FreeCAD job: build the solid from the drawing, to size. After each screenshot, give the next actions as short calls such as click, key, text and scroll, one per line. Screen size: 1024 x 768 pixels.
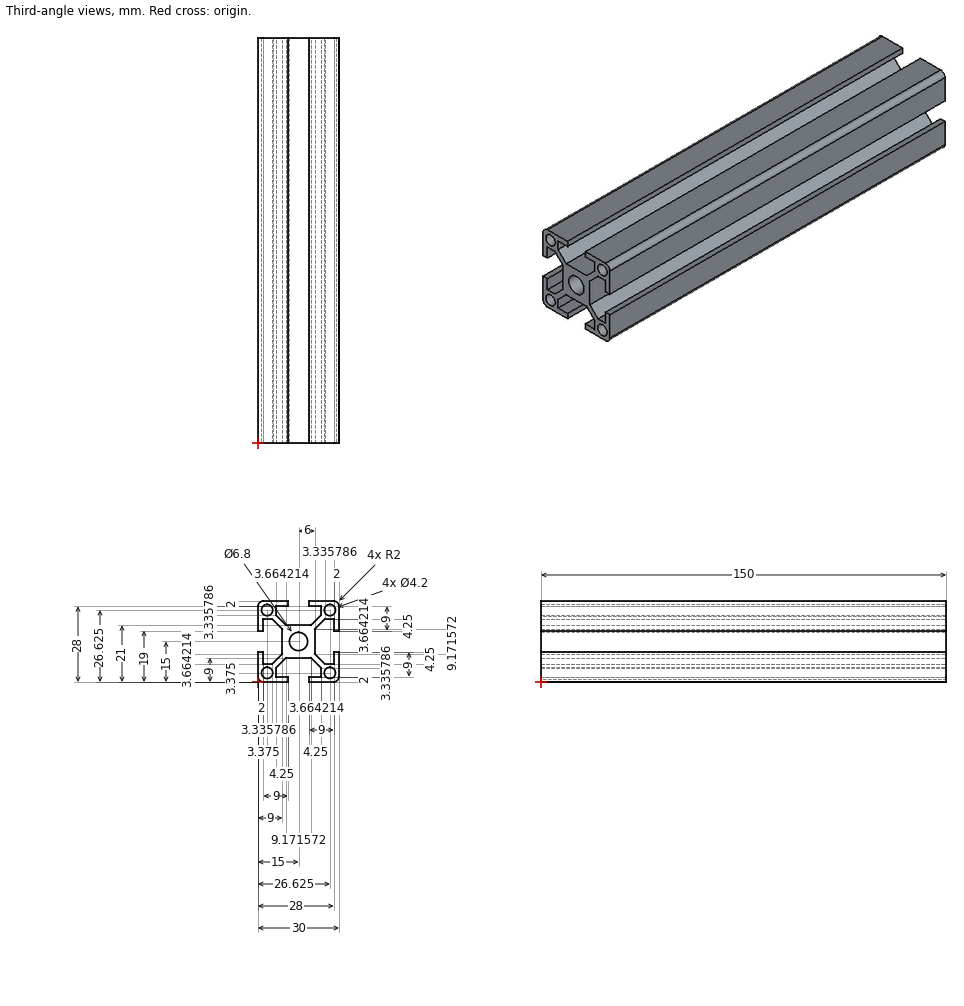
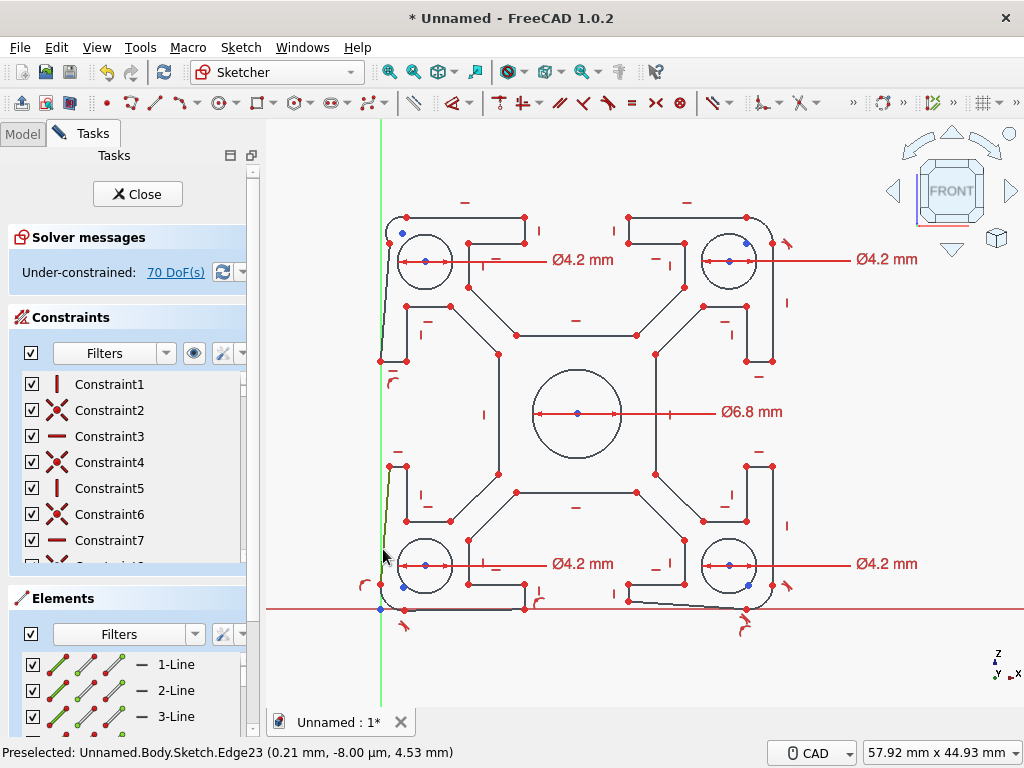
click(382, 596)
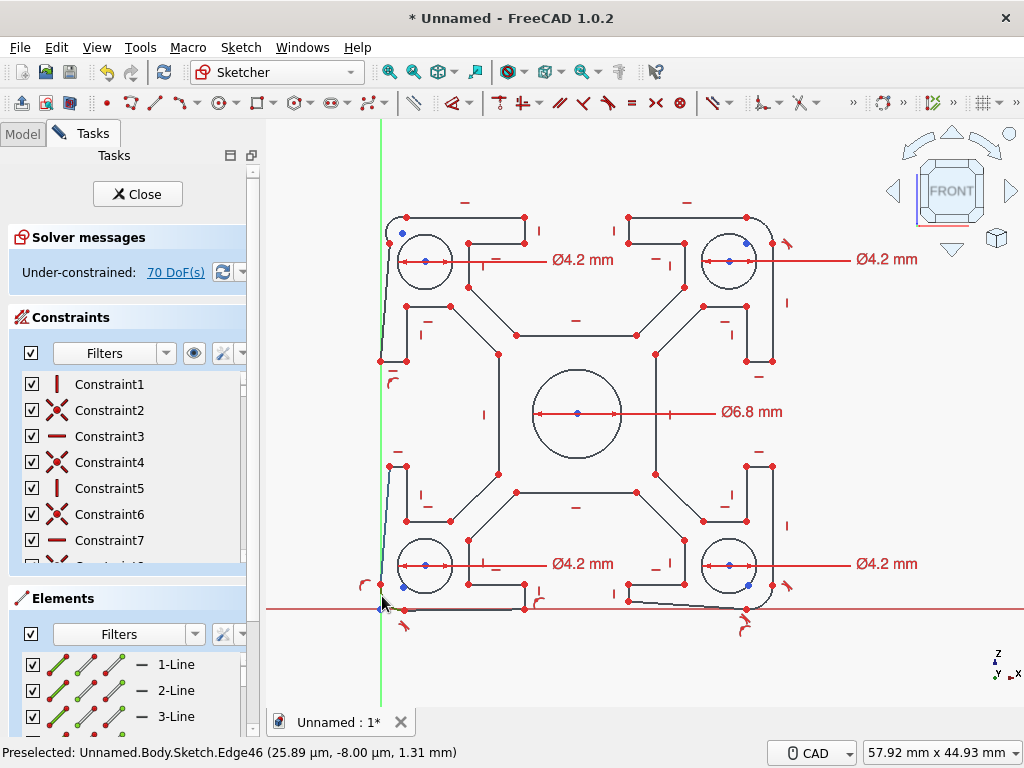
key(t)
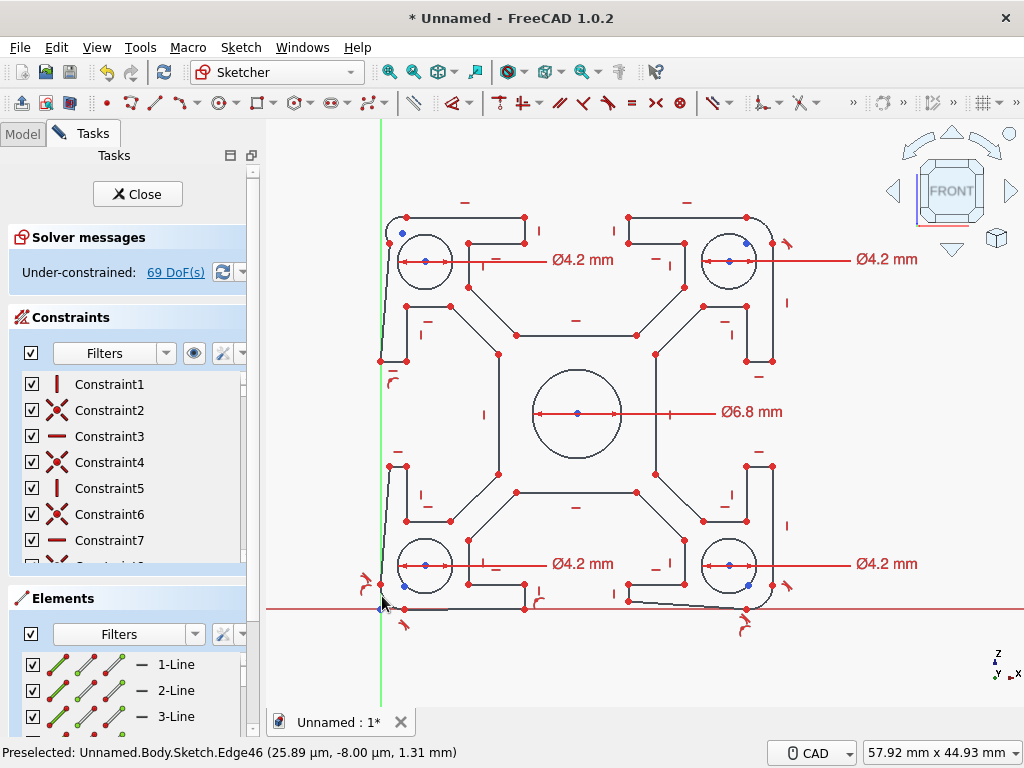
click(383, 326)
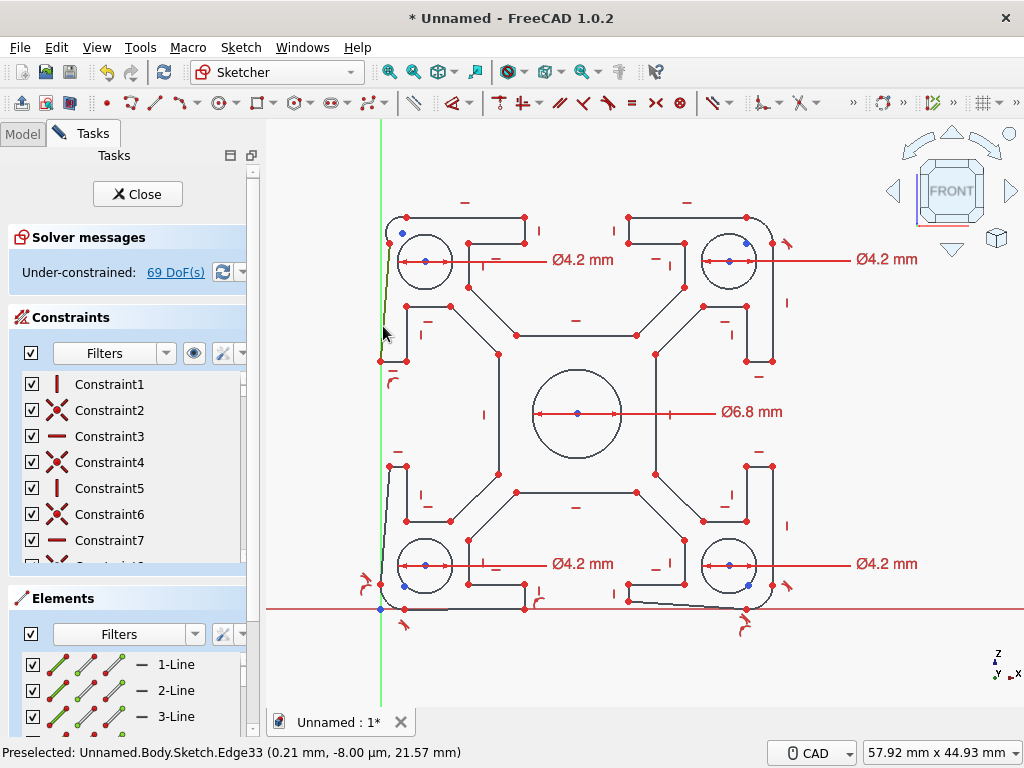
click(395, 219)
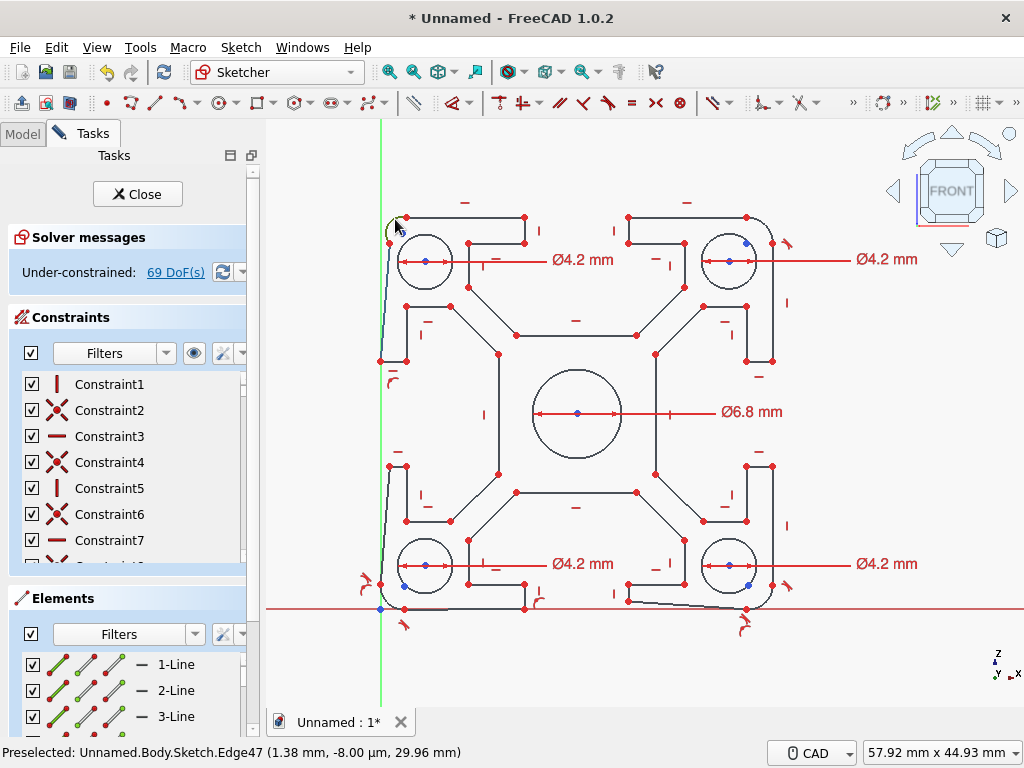
key(t)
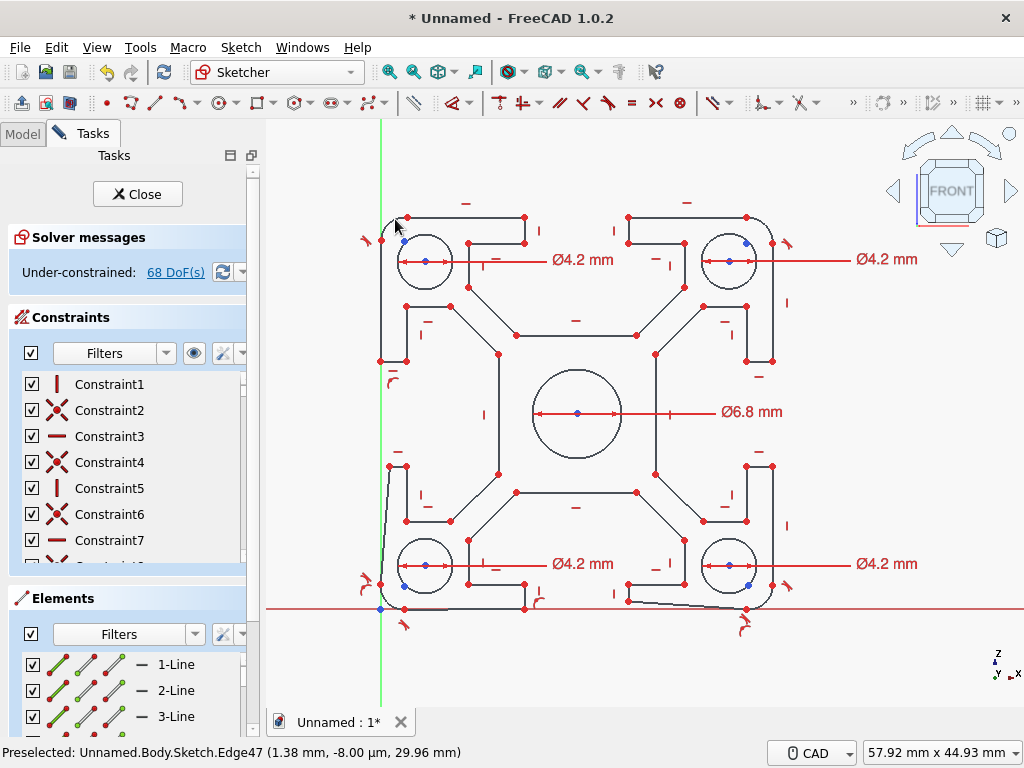
click(442, 218)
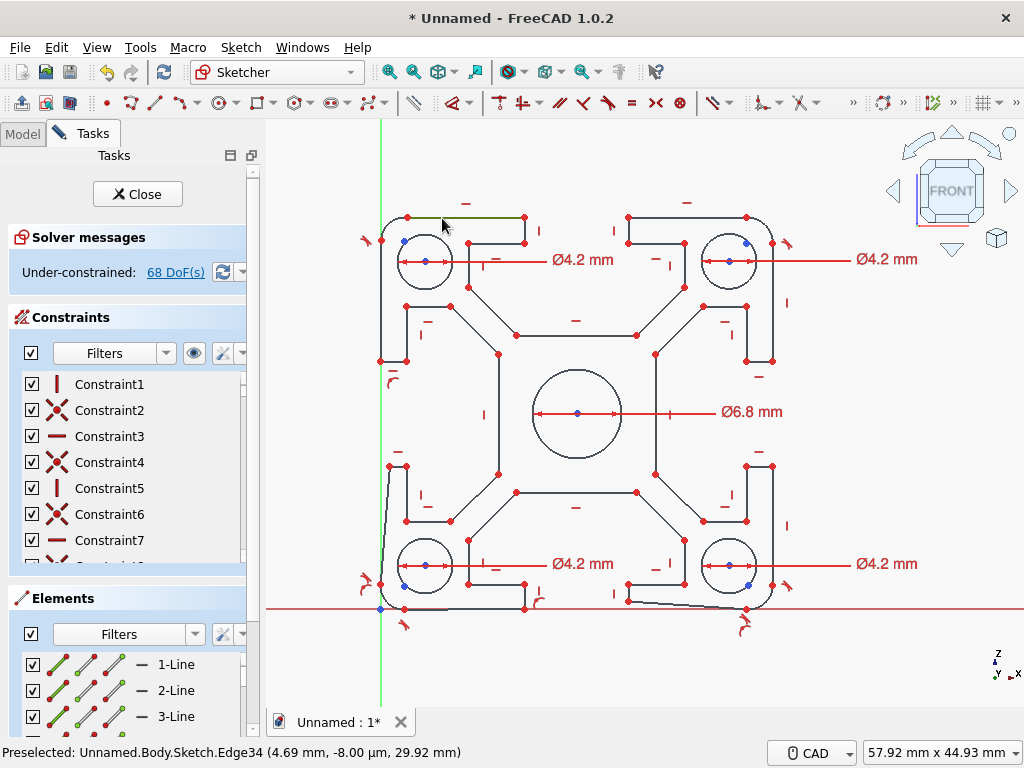
click(396, 219)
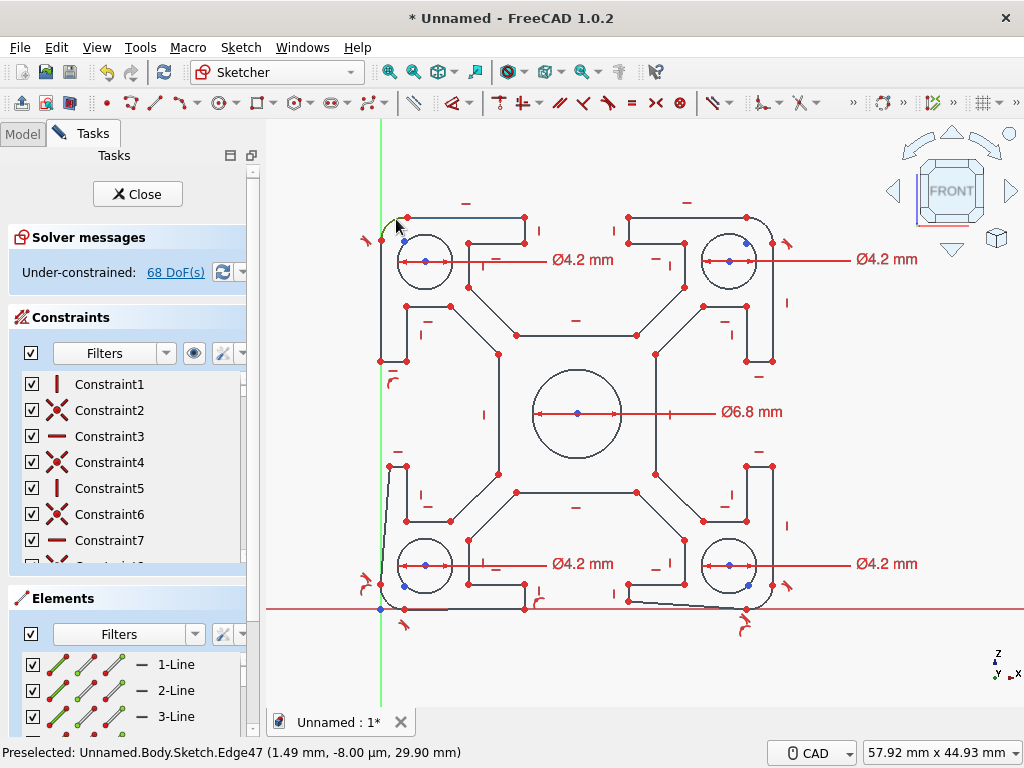
key(t)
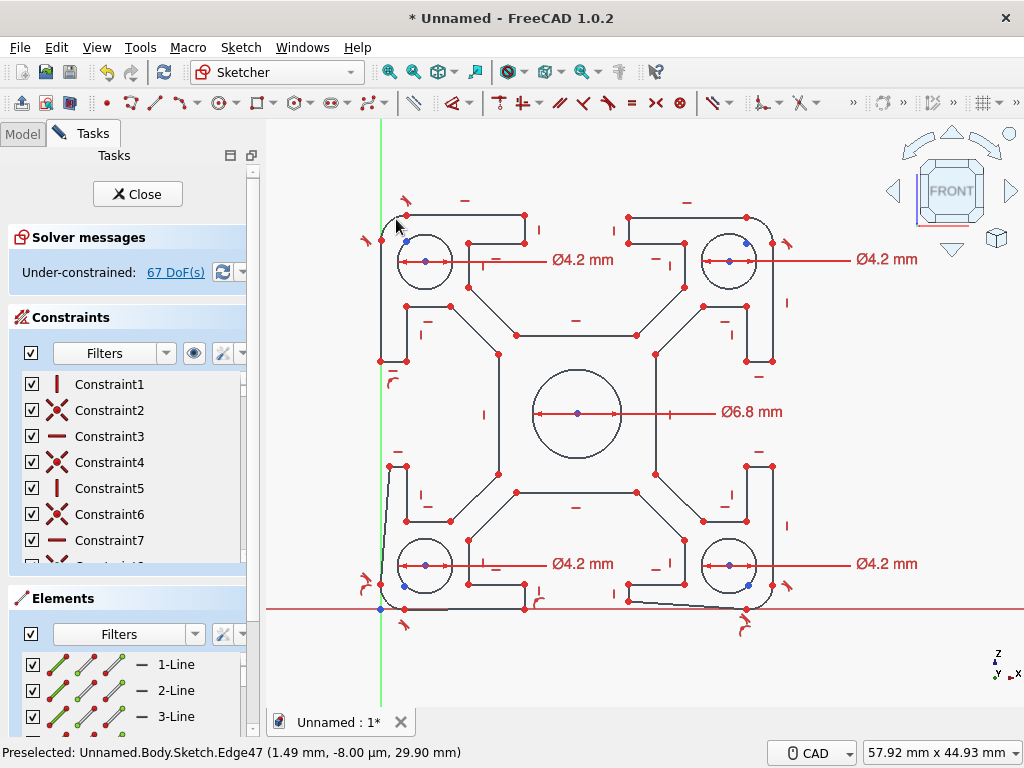
click(664, 218)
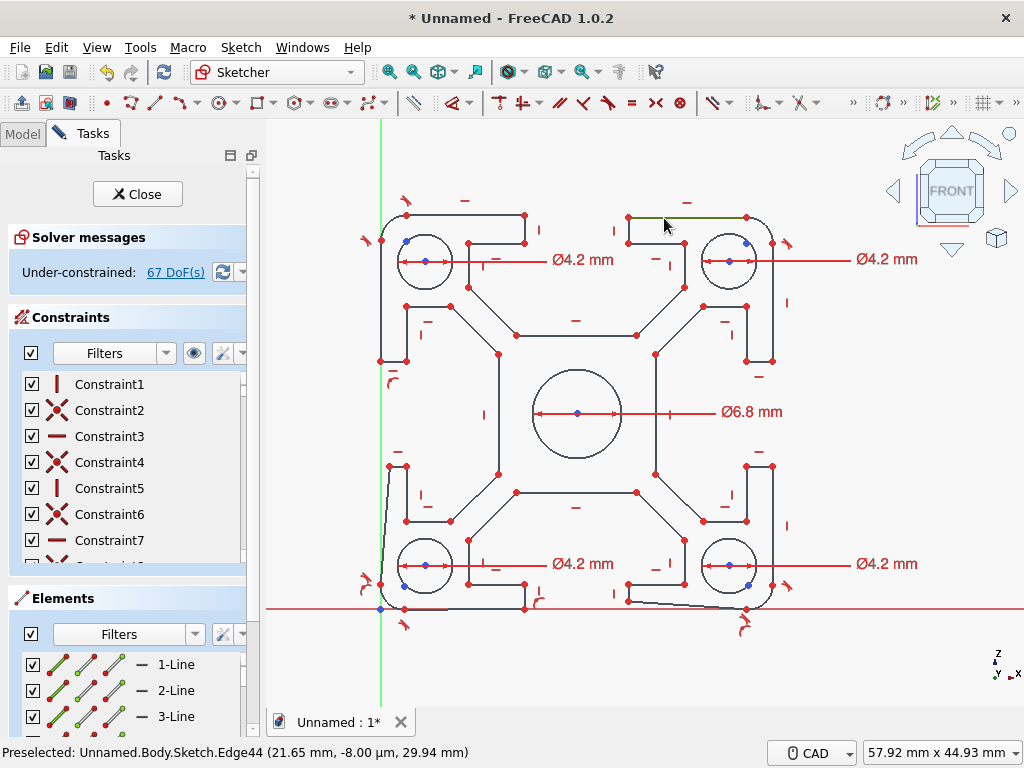
click(770, 232)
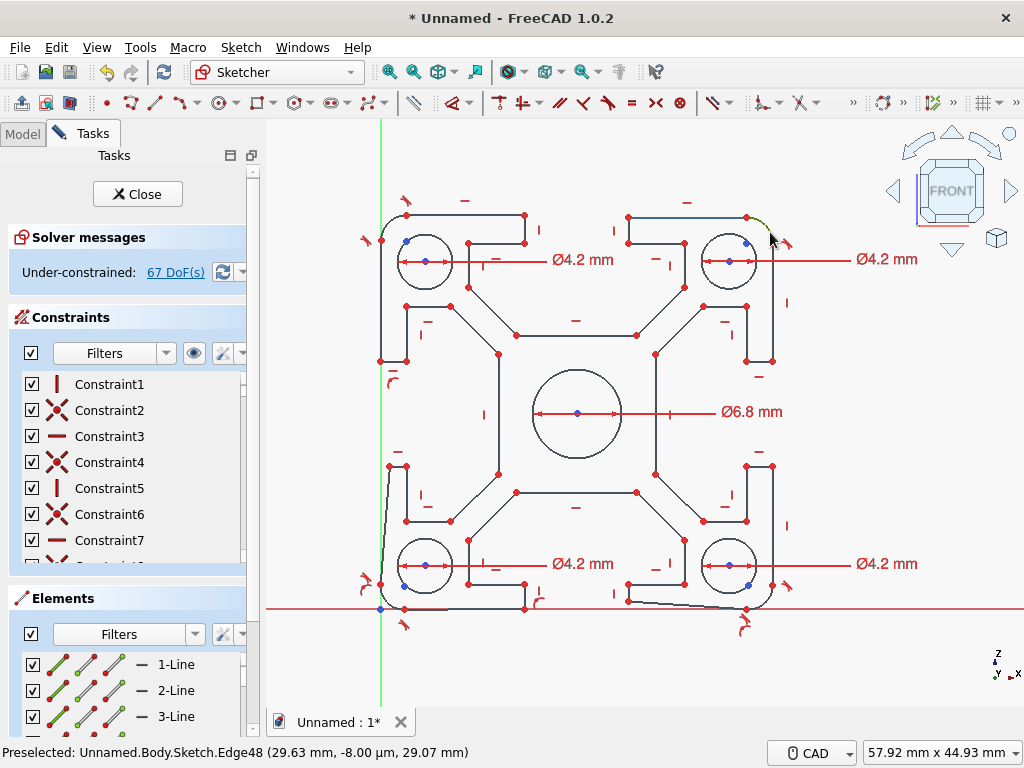
key(t)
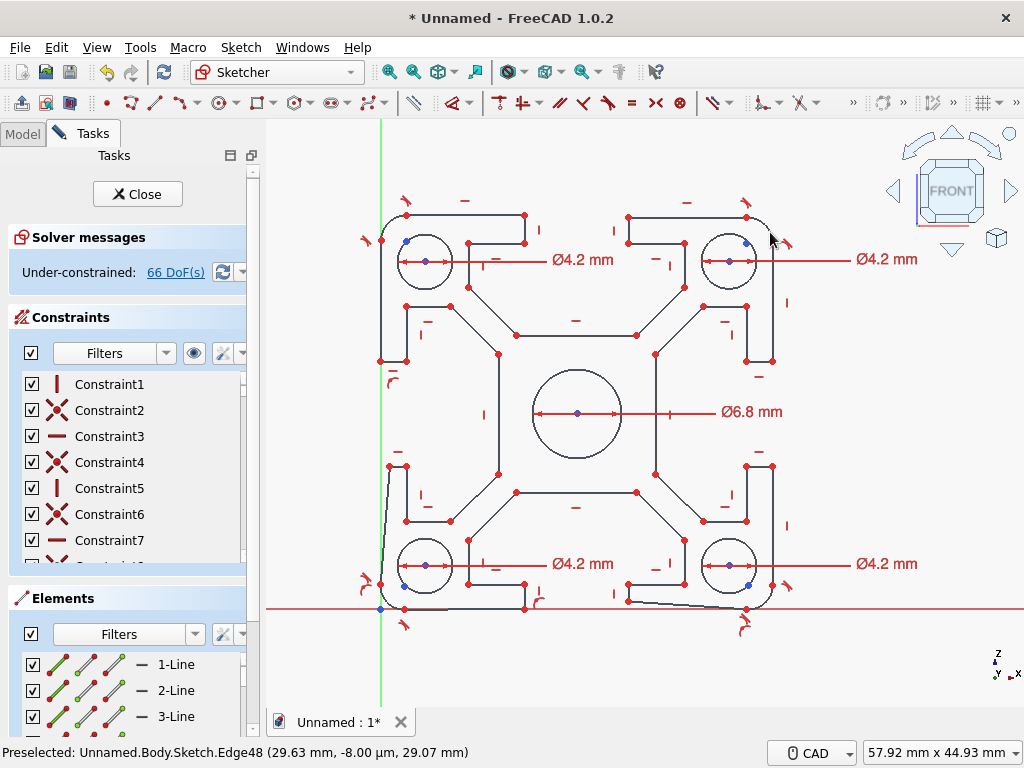
click(711, 607)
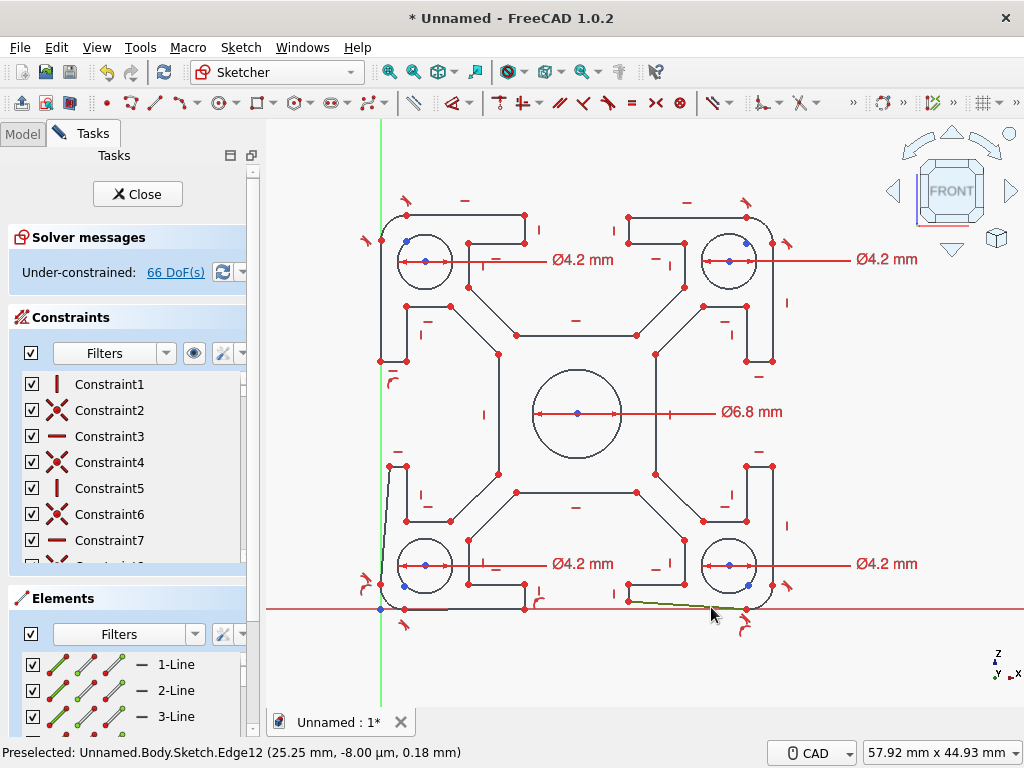
key(h)